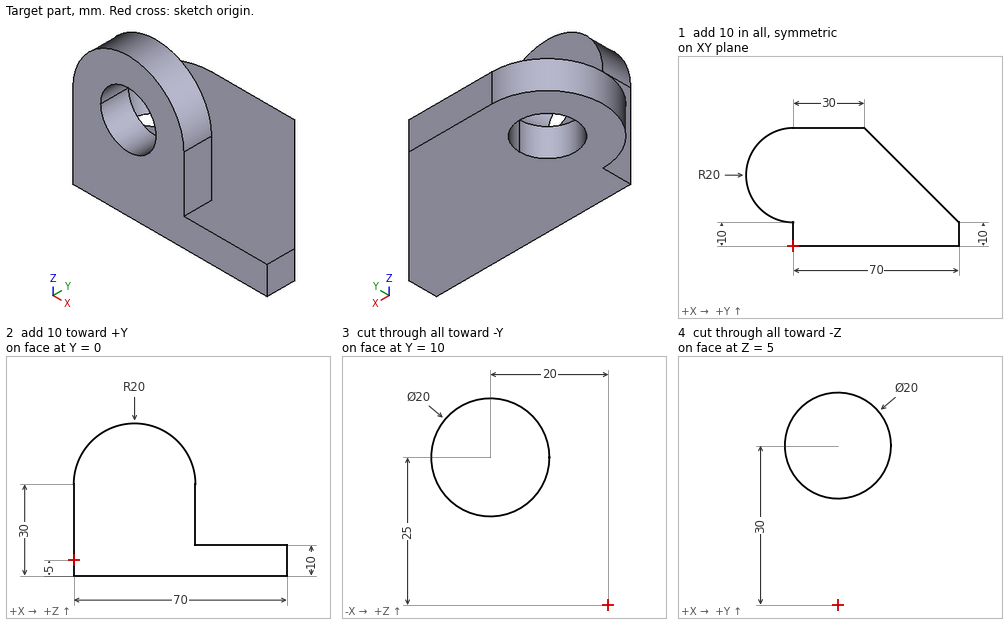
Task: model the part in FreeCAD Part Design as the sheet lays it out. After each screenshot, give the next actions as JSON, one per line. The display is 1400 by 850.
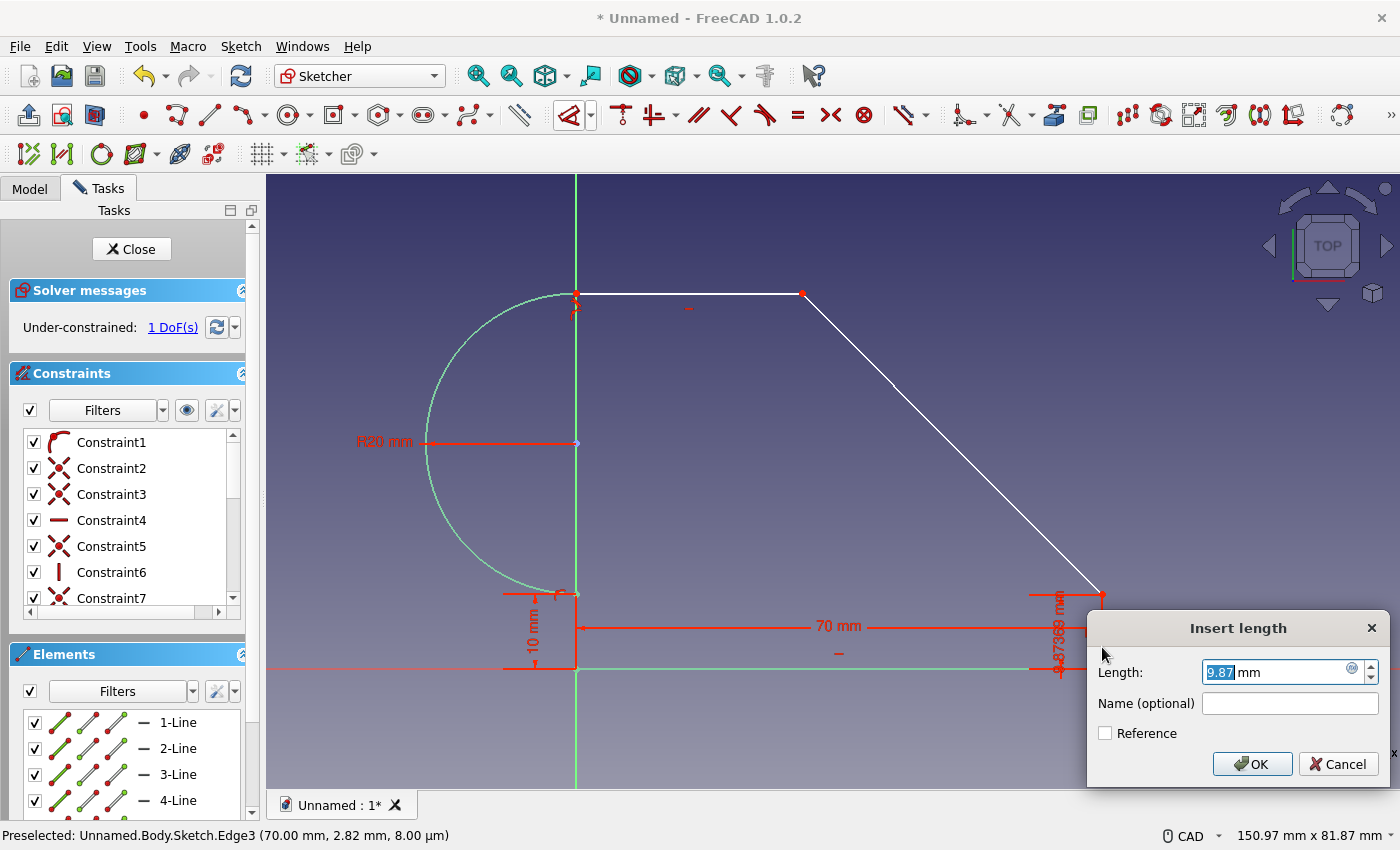
{"action": "type", "text": "10"}
{"action": "key", "text": "Return"}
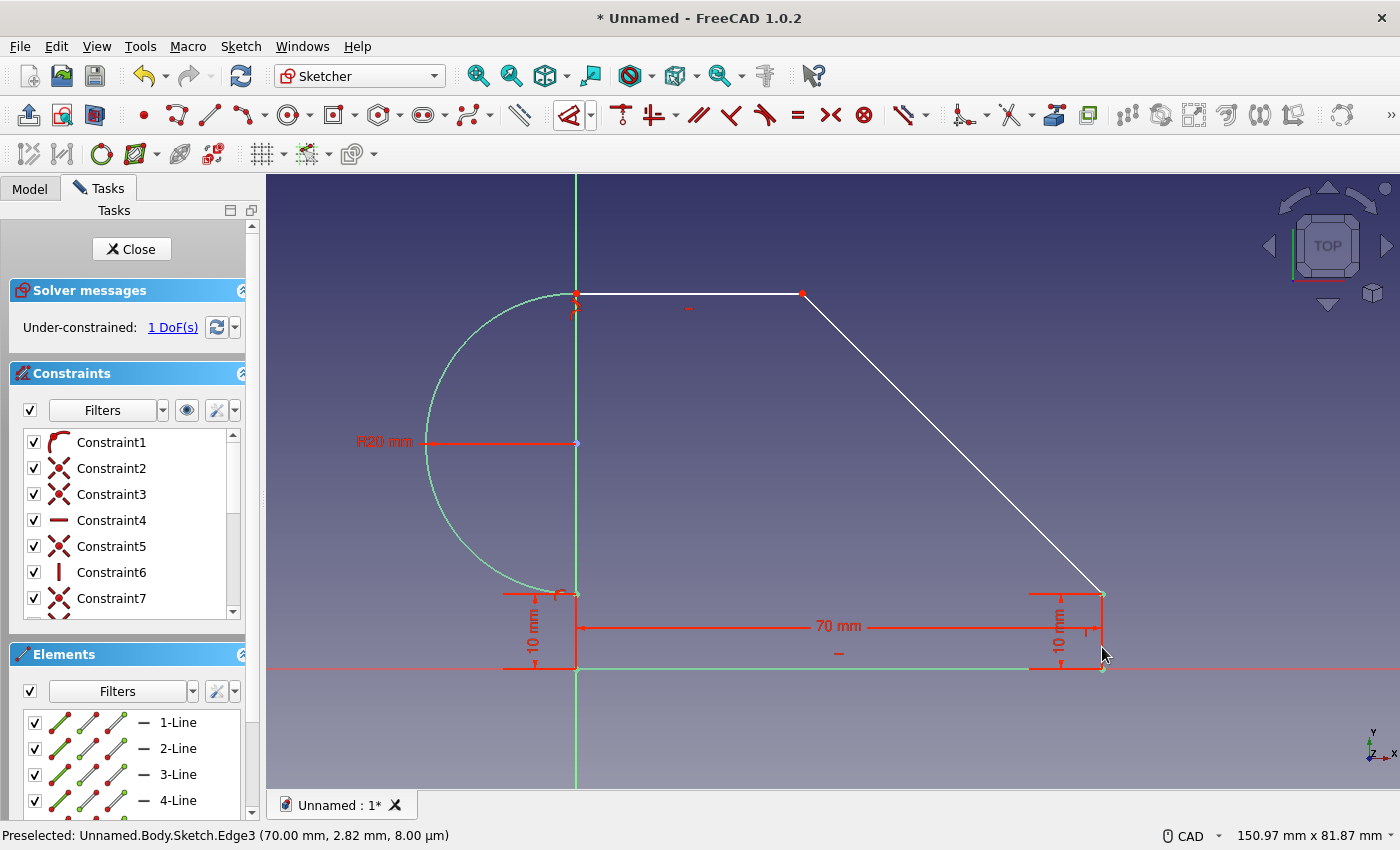
{"action": "left_click", "coordinate": [734, 294]}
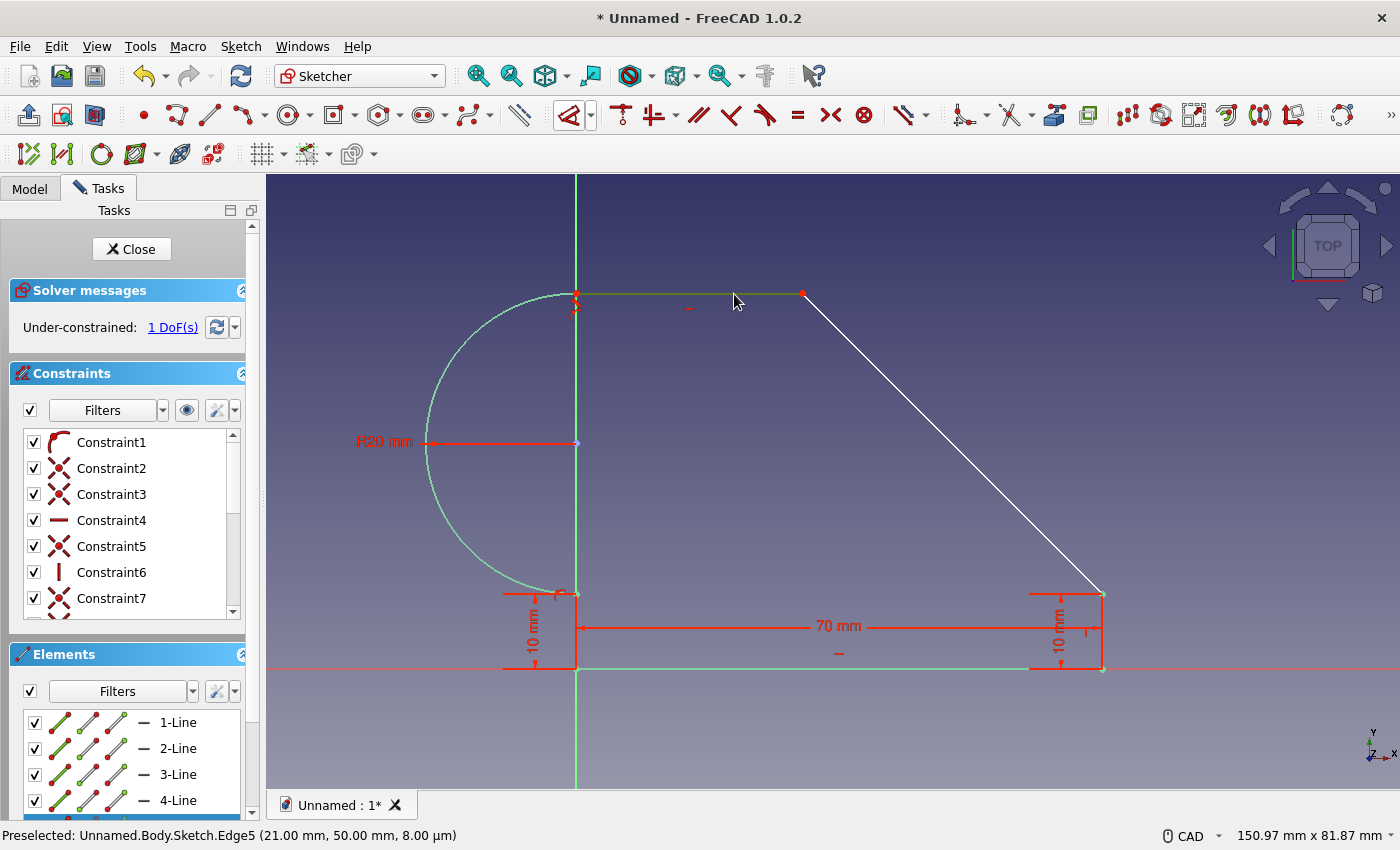
{"action": "left_click", "coordinate": [590, 116]}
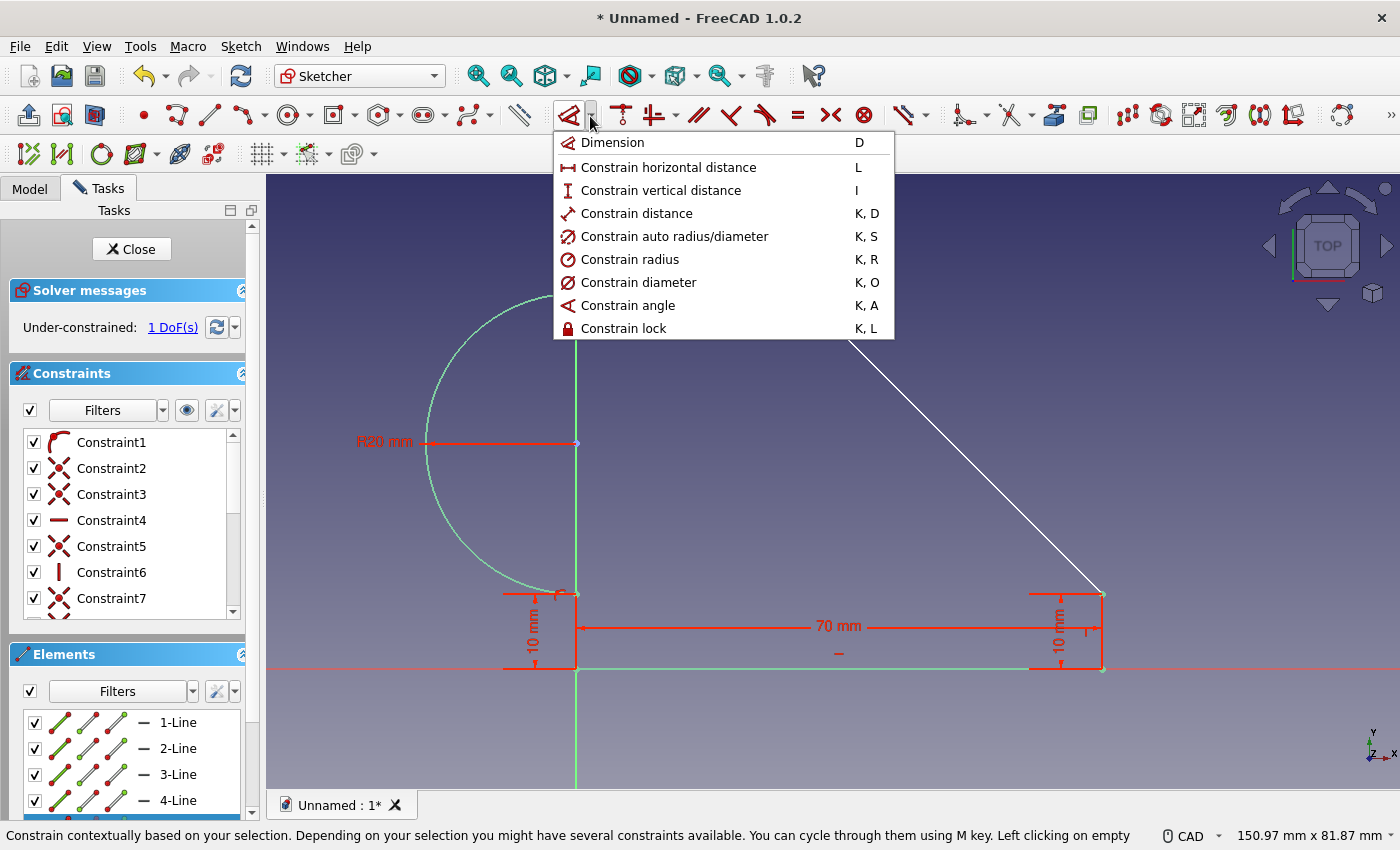
{"action": "left_click", "coordinate": [724, 168]}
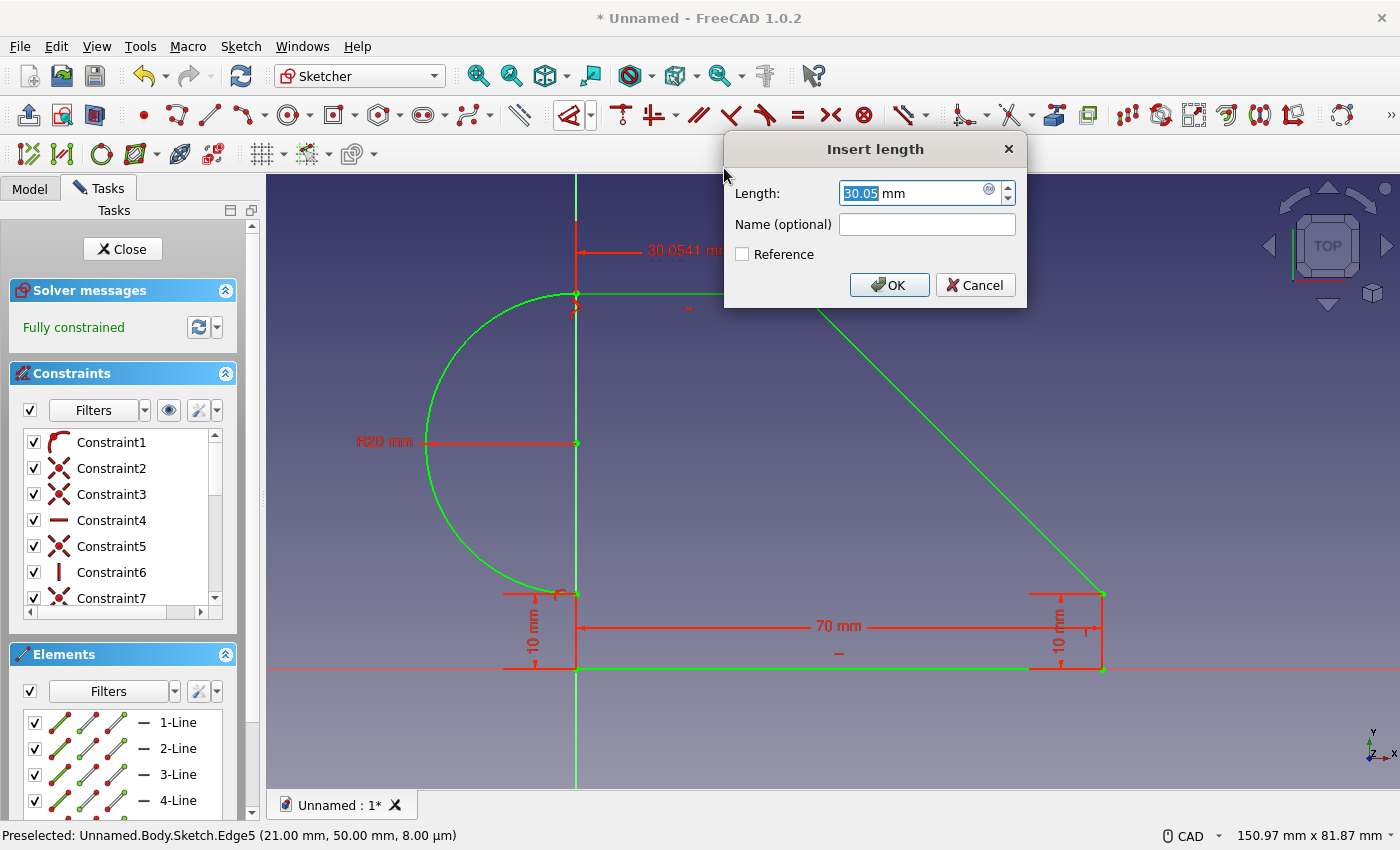
{"action": "type", "text": "30"}
{"action": "key", "text": "Return"}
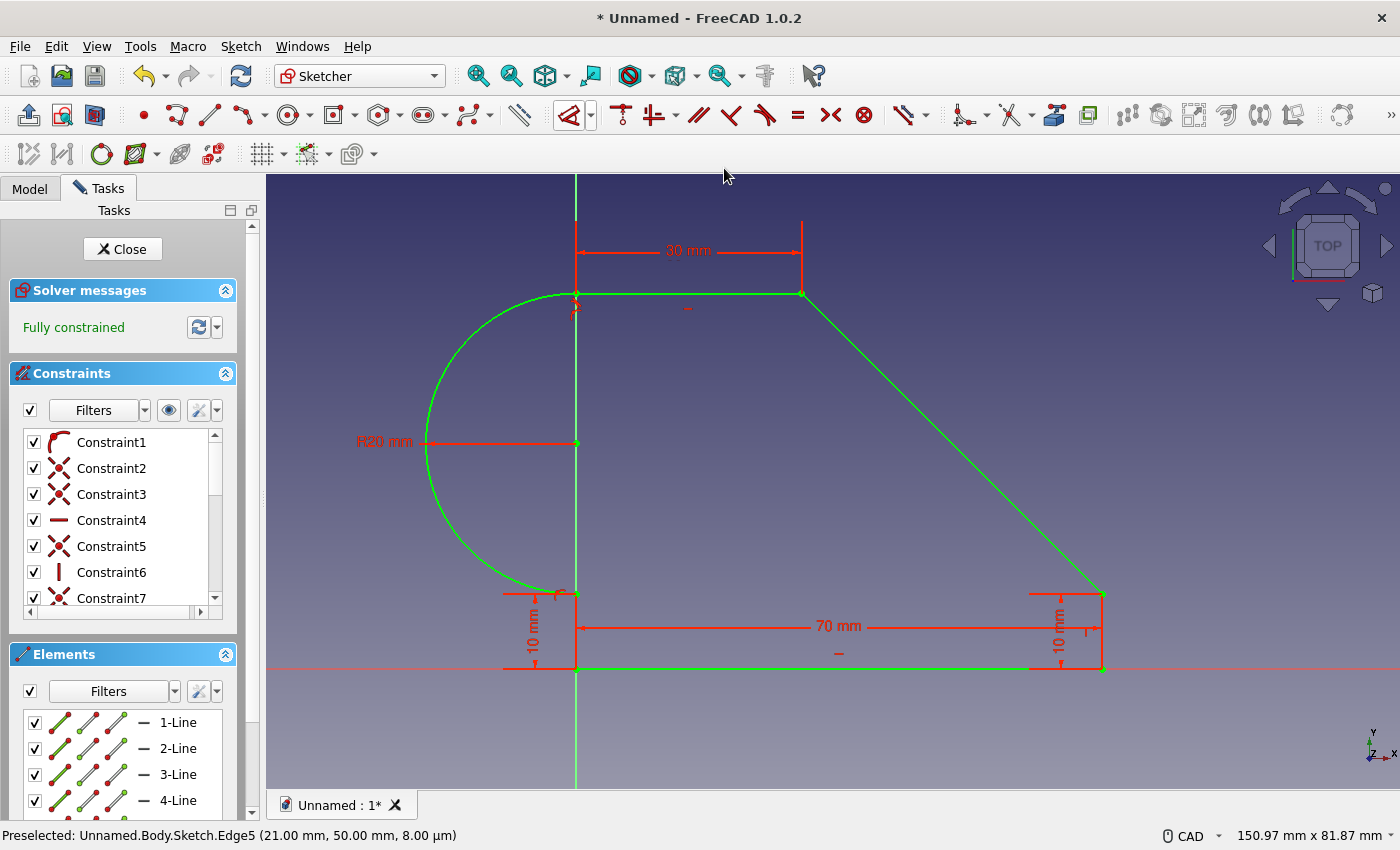
{"action": "left_click", "coordinate": [123, 249]}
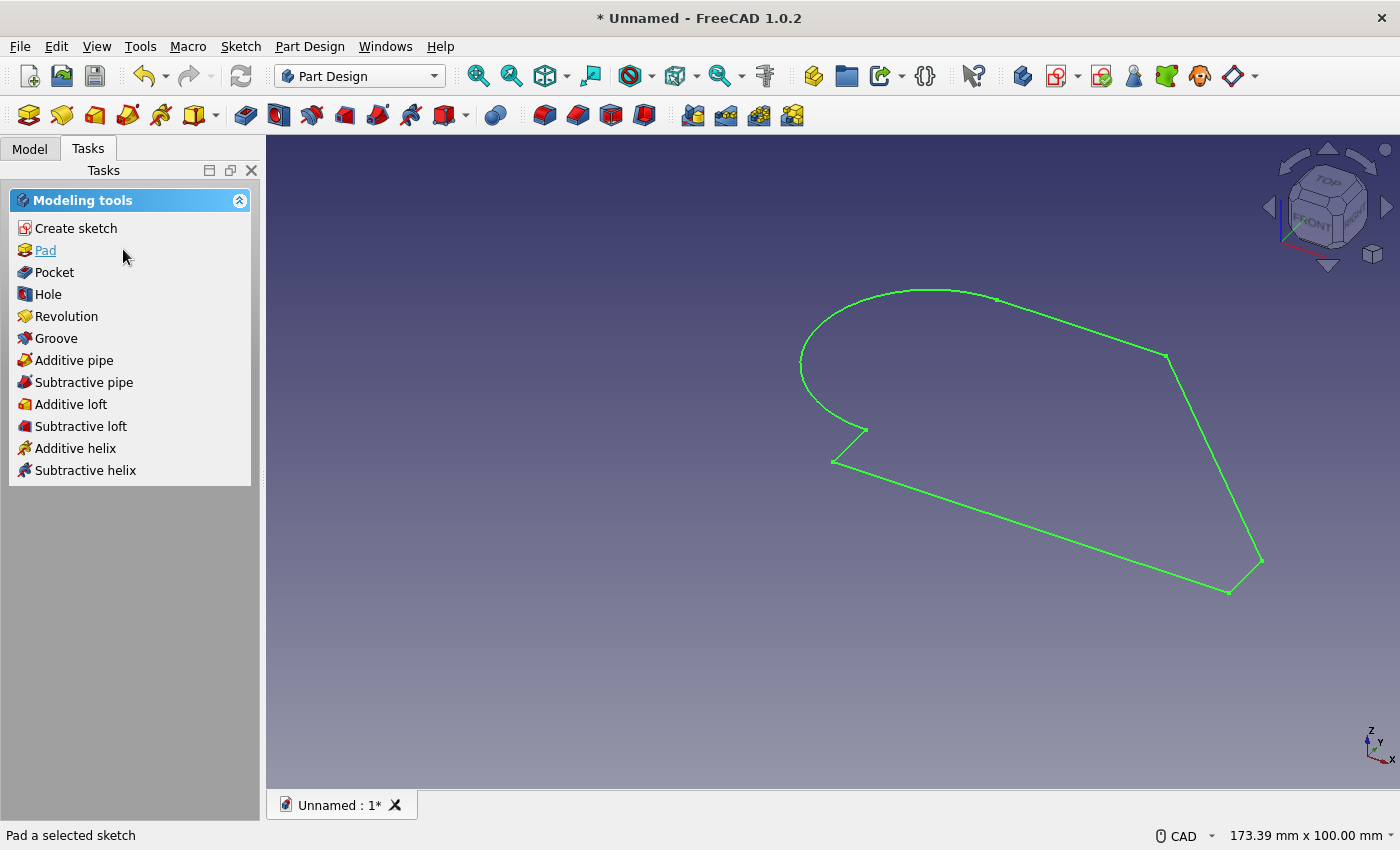
{"action": "left_click", "coordinate": [29, 116]}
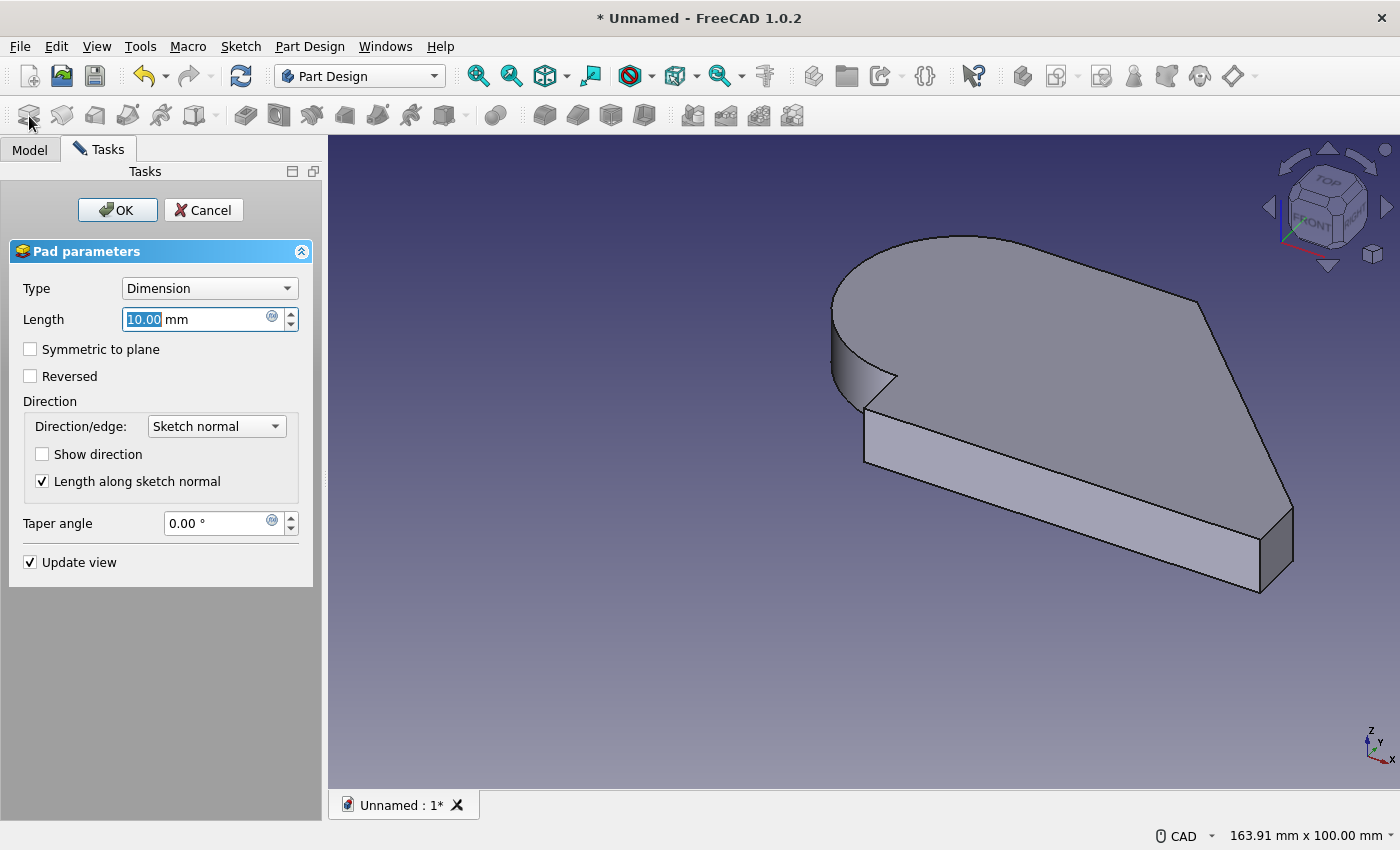
{"action": "type", "text": "10"}
{"action": "key", "text": "Tab"}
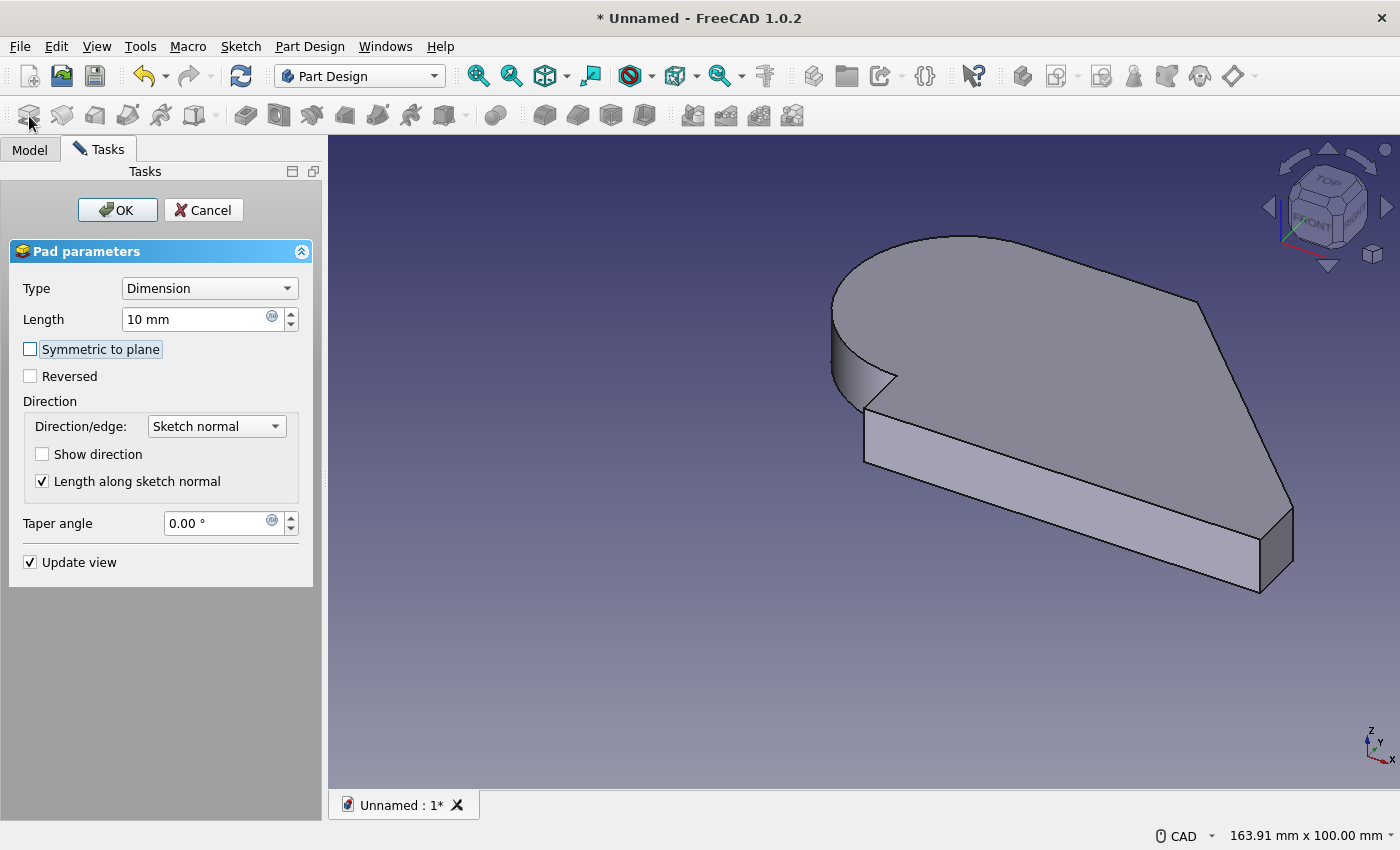
{"action": "left_click", "coordinate": [31, 349]}